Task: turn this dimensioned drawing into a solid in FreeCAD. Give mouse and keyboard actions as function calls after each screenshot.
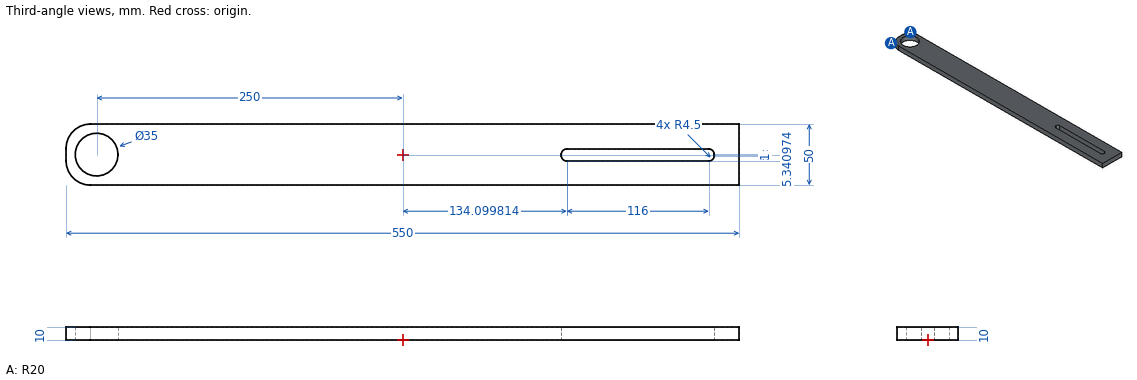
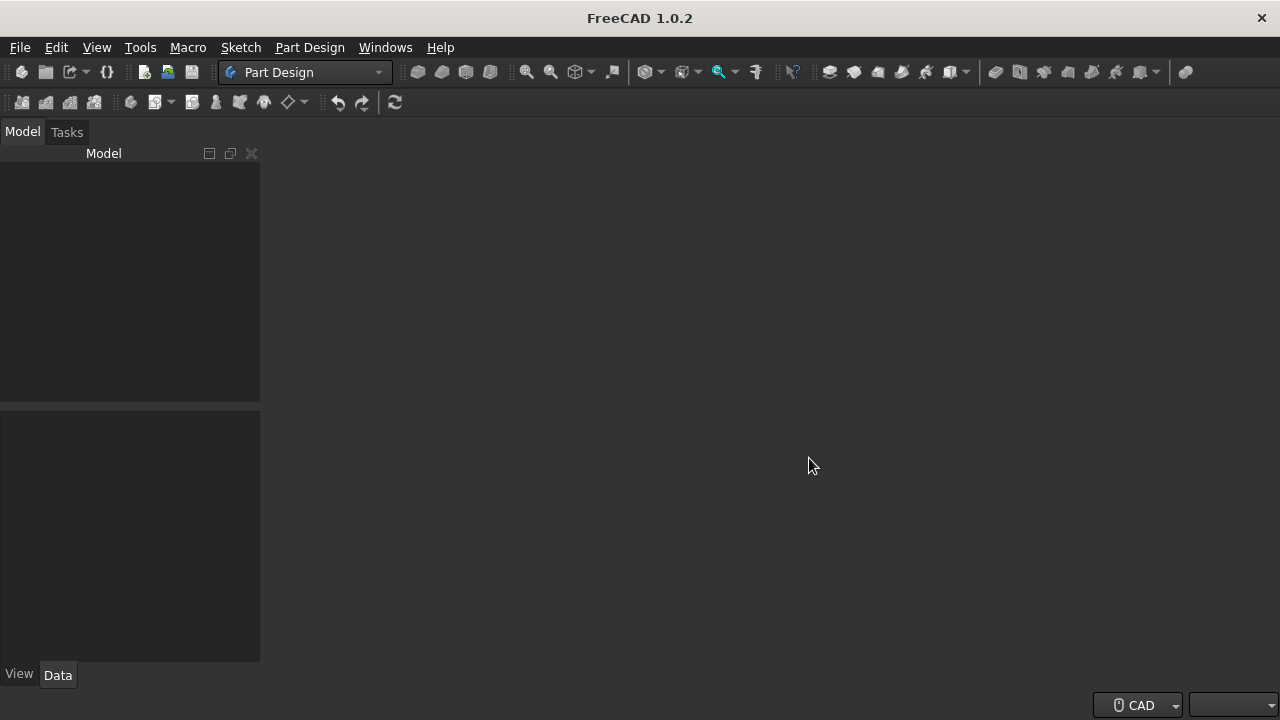
click(144, 72)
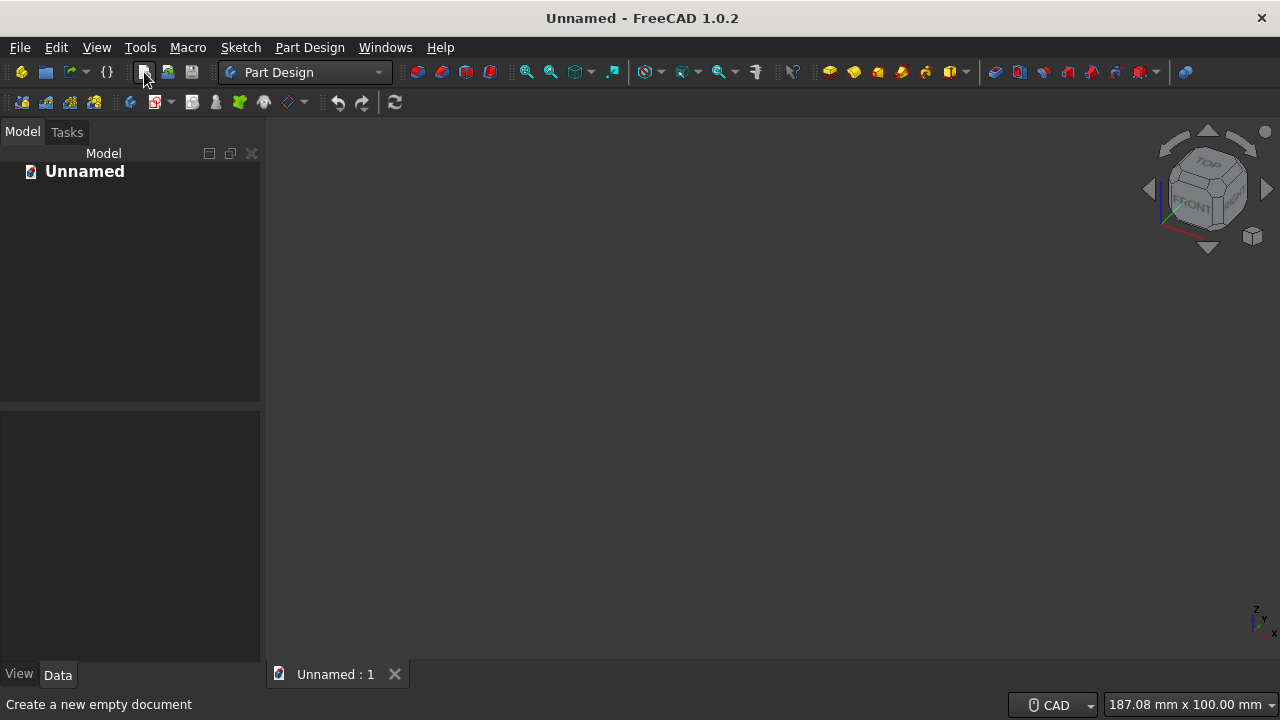
click(156, 102)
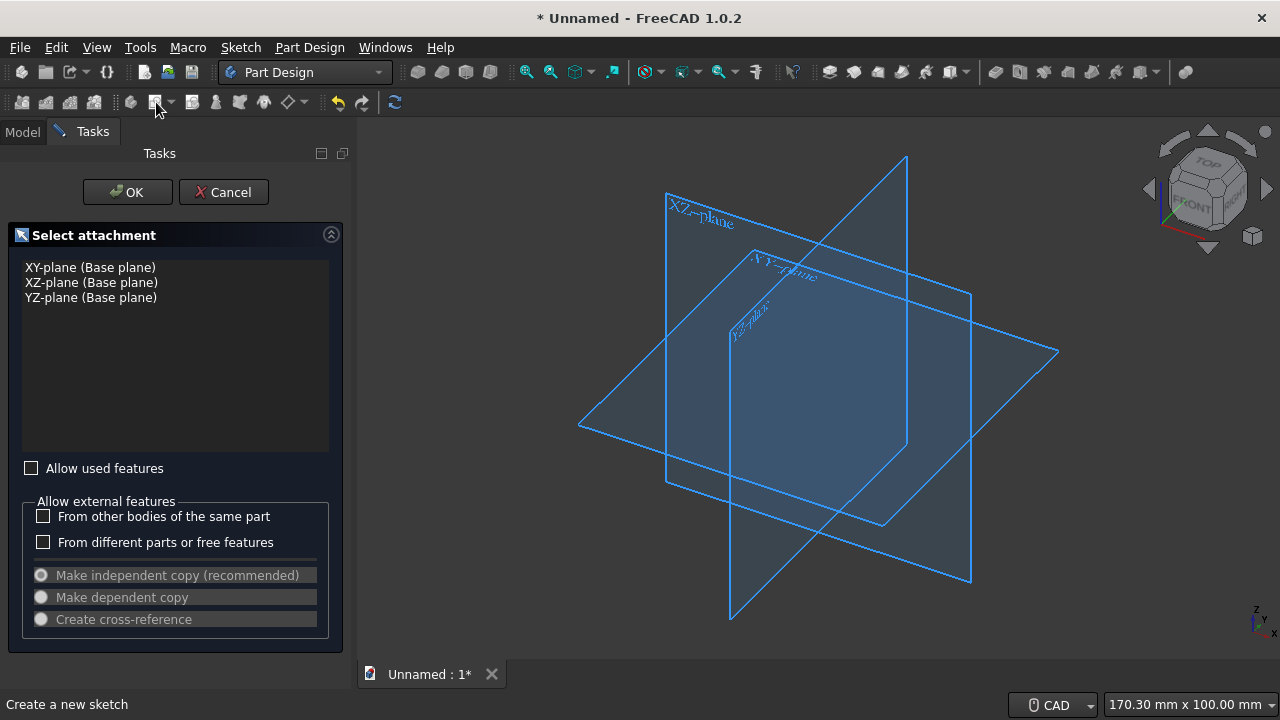
click(82, 268)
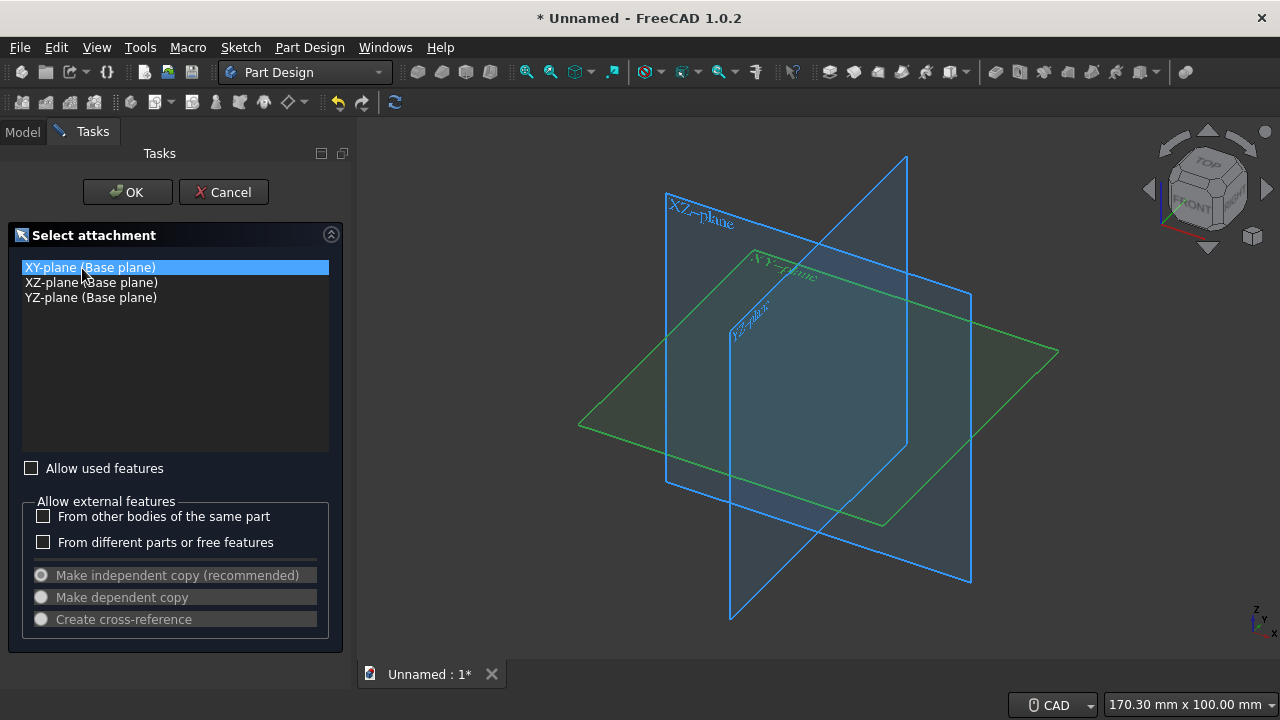
click(128, 192)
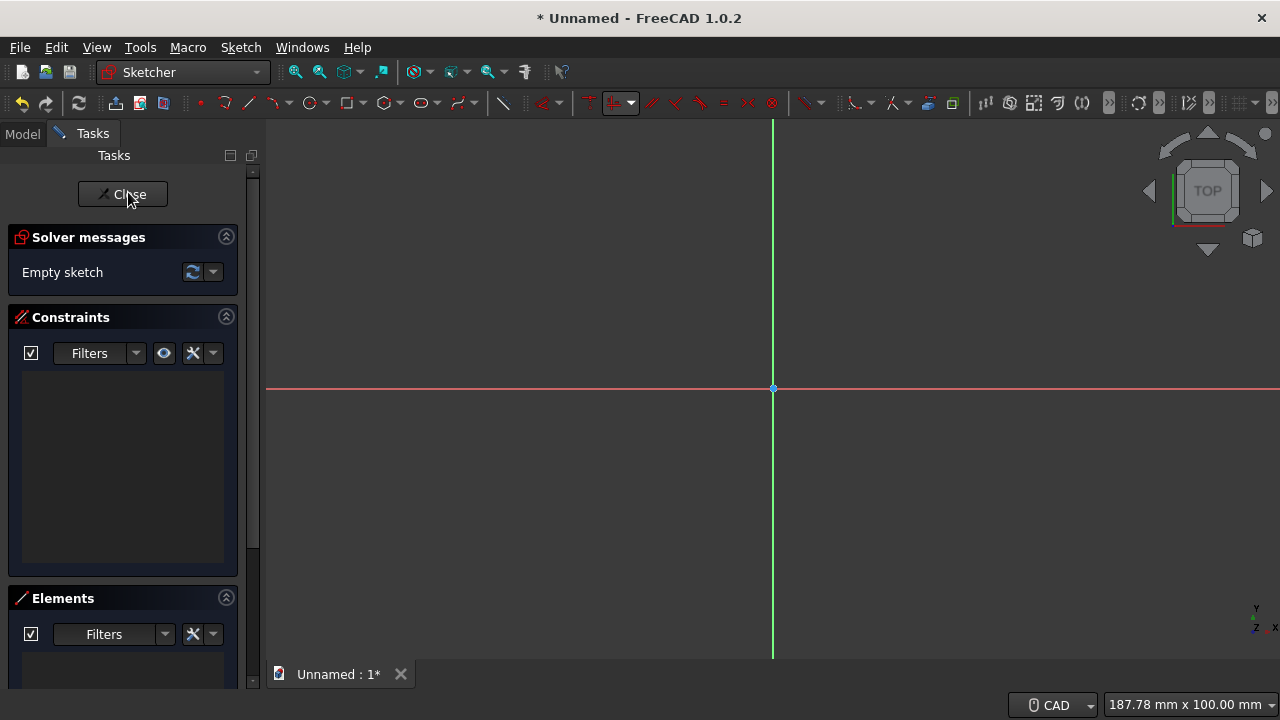
scroll(687, 389, down, 8)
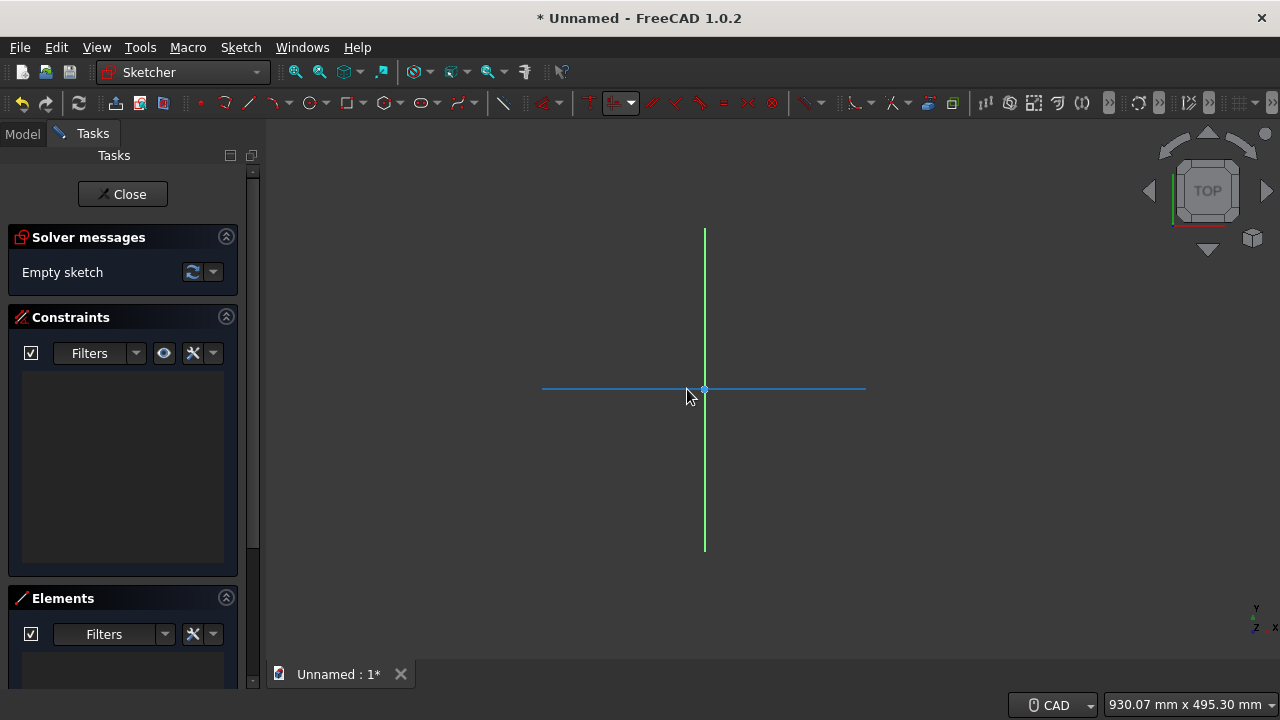
key(g)
key(v)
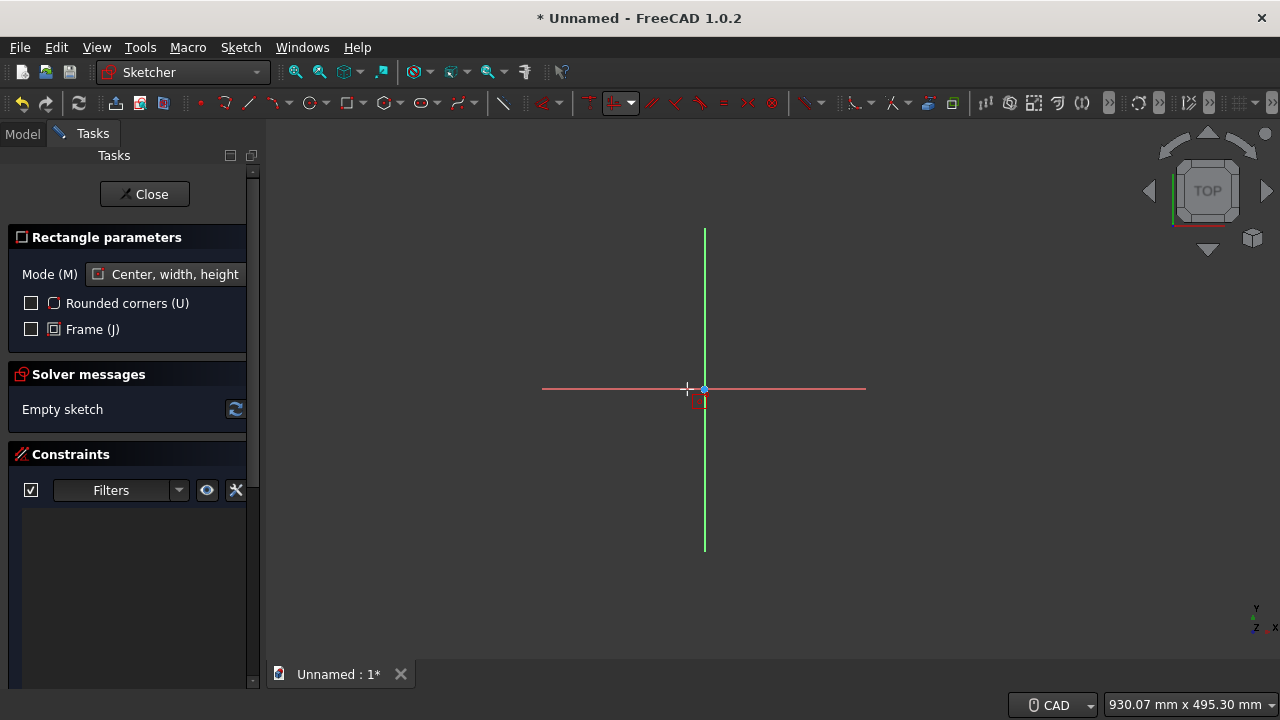
click(705, 389)
click(1005, 362)
key(Escape)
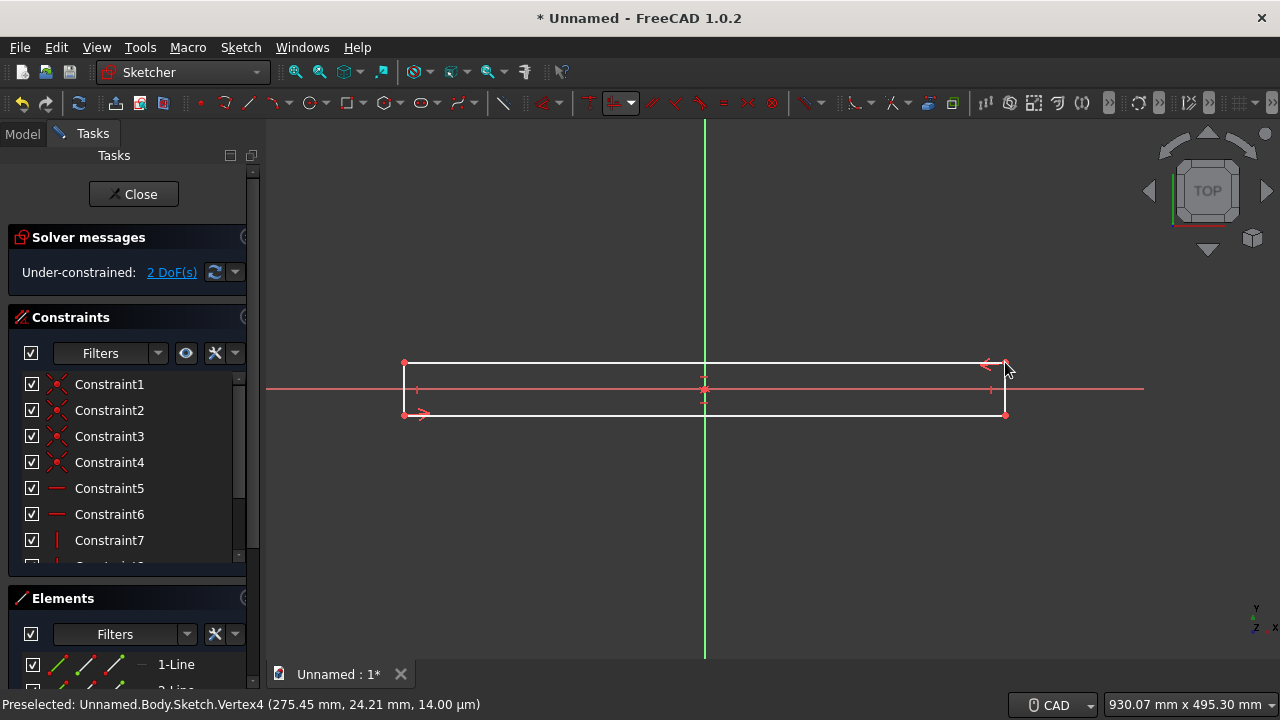
scroll(1005, 400, up, 2)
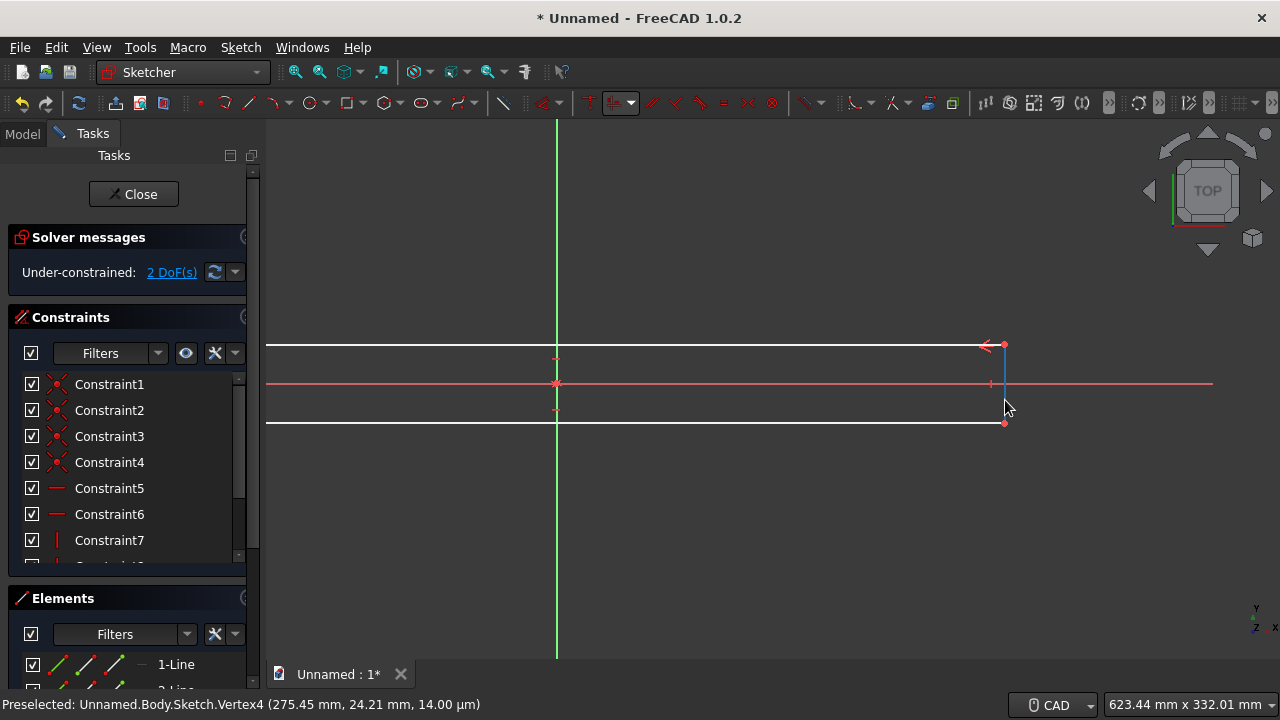
click(1005, 400)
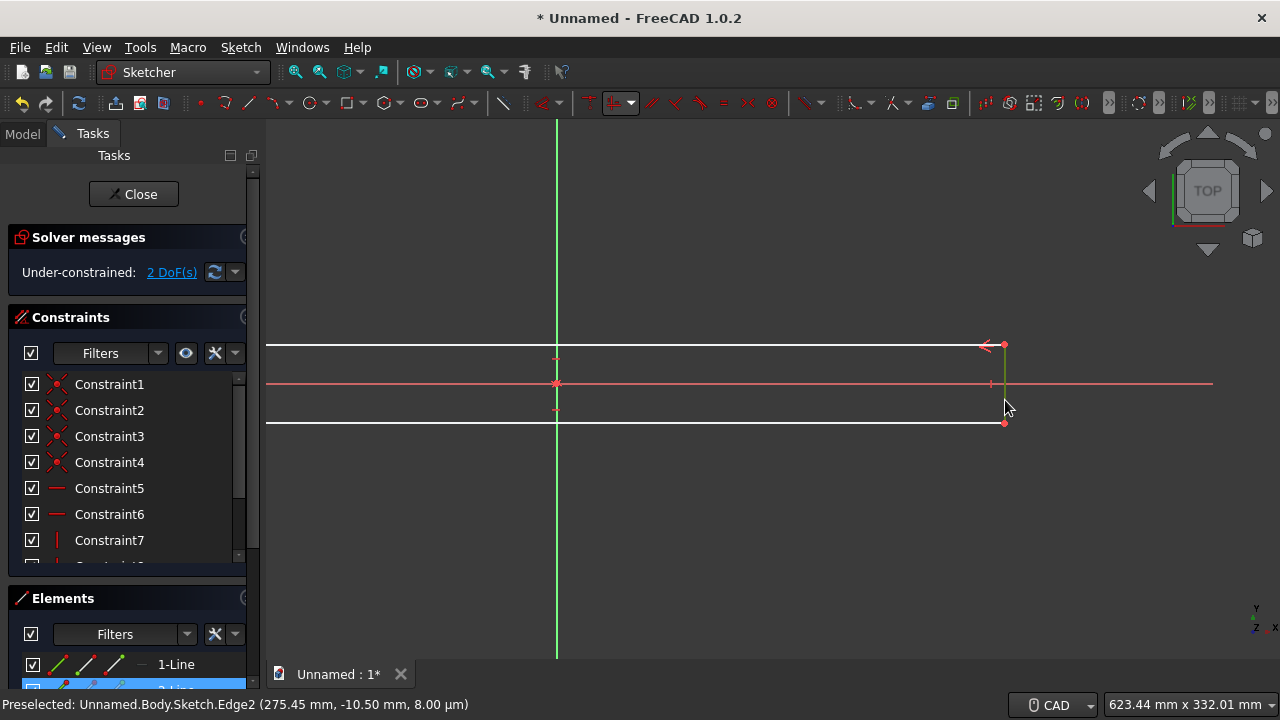
click(562, 104)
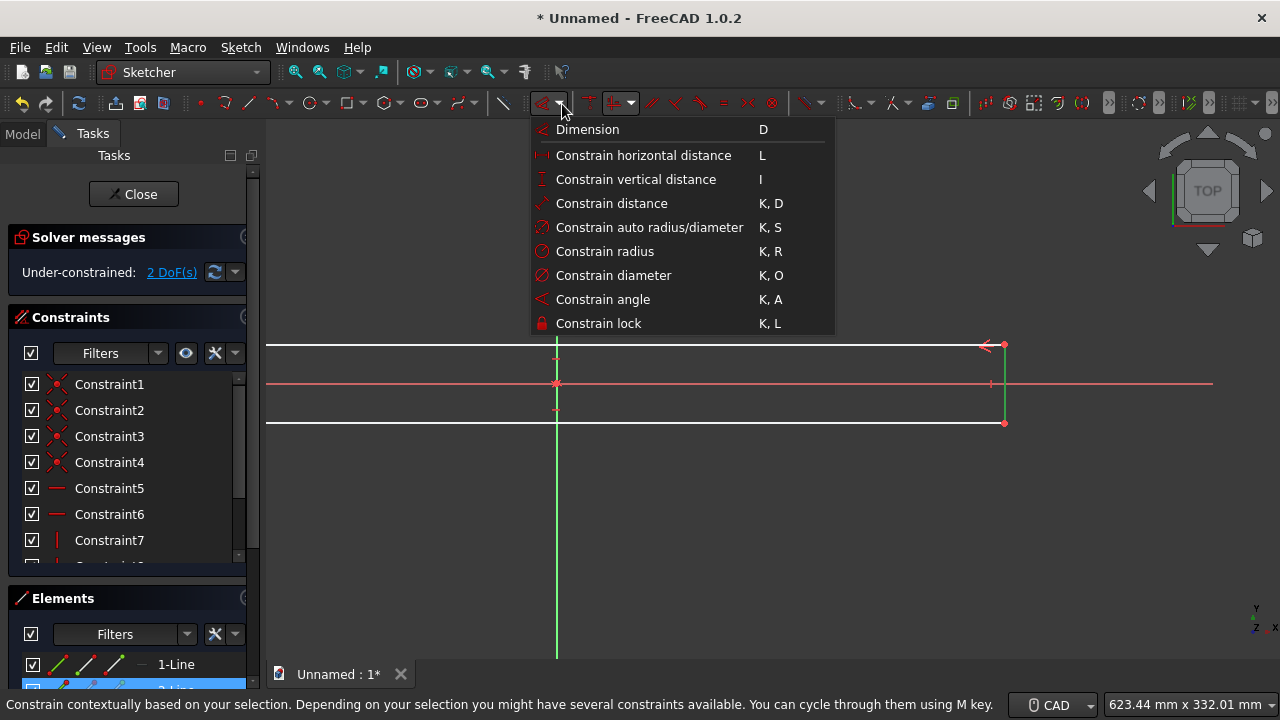
click(683, 179)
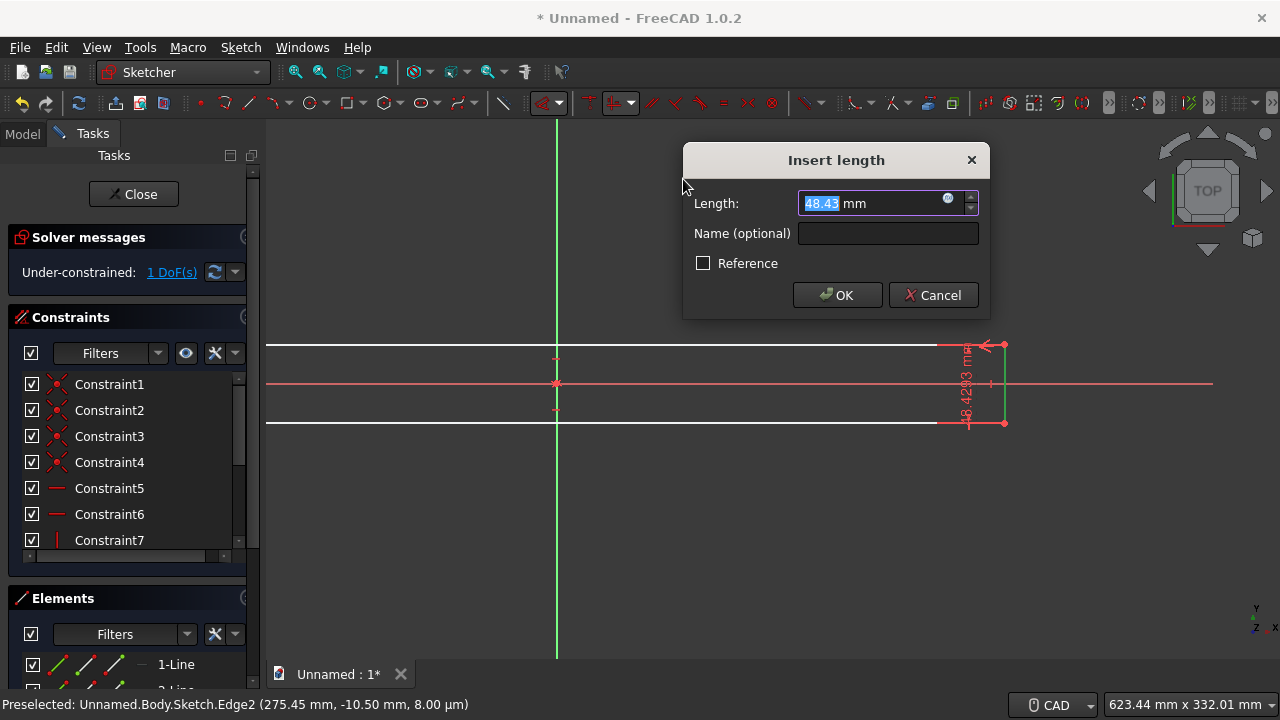
text(50)
key(Return)